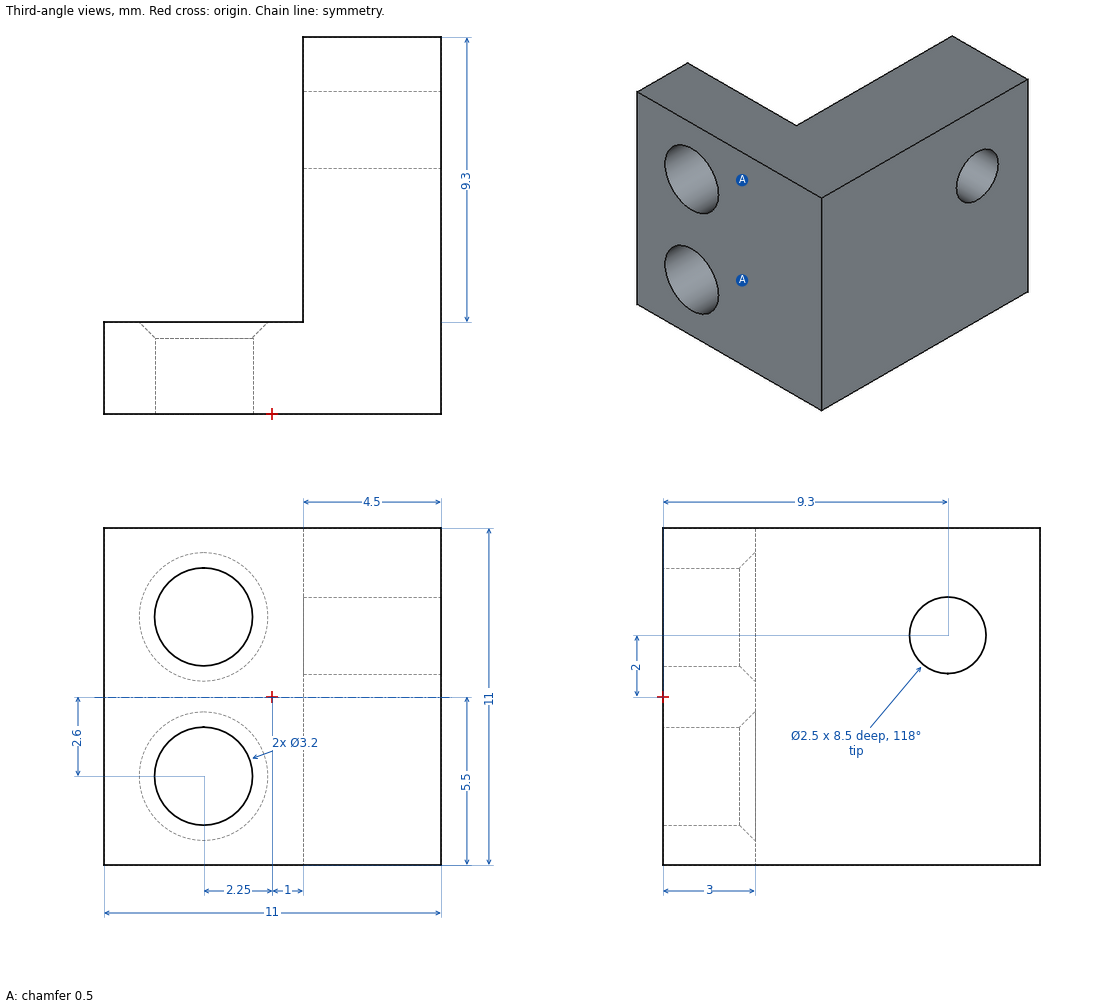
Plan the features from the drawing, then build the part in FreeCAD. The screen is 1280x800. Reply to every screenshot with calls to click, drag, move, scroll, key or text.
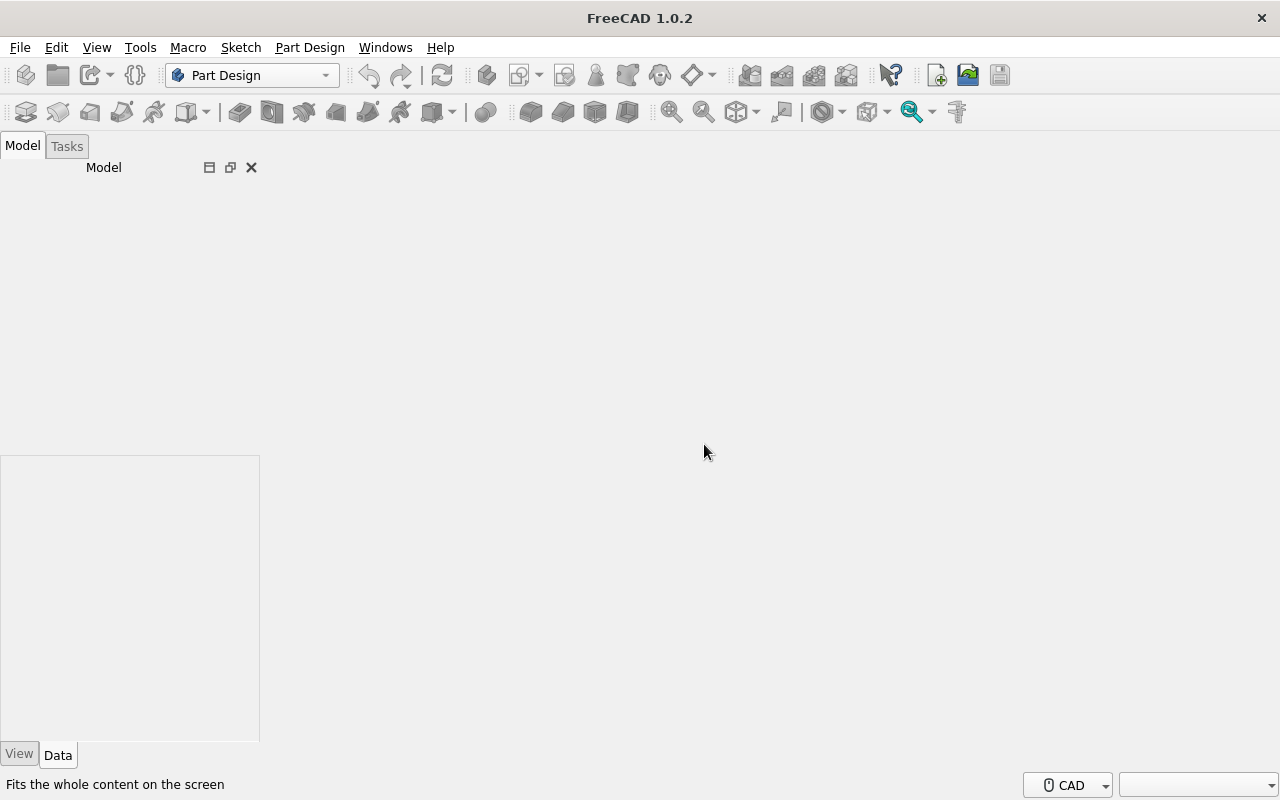
click(936, 76)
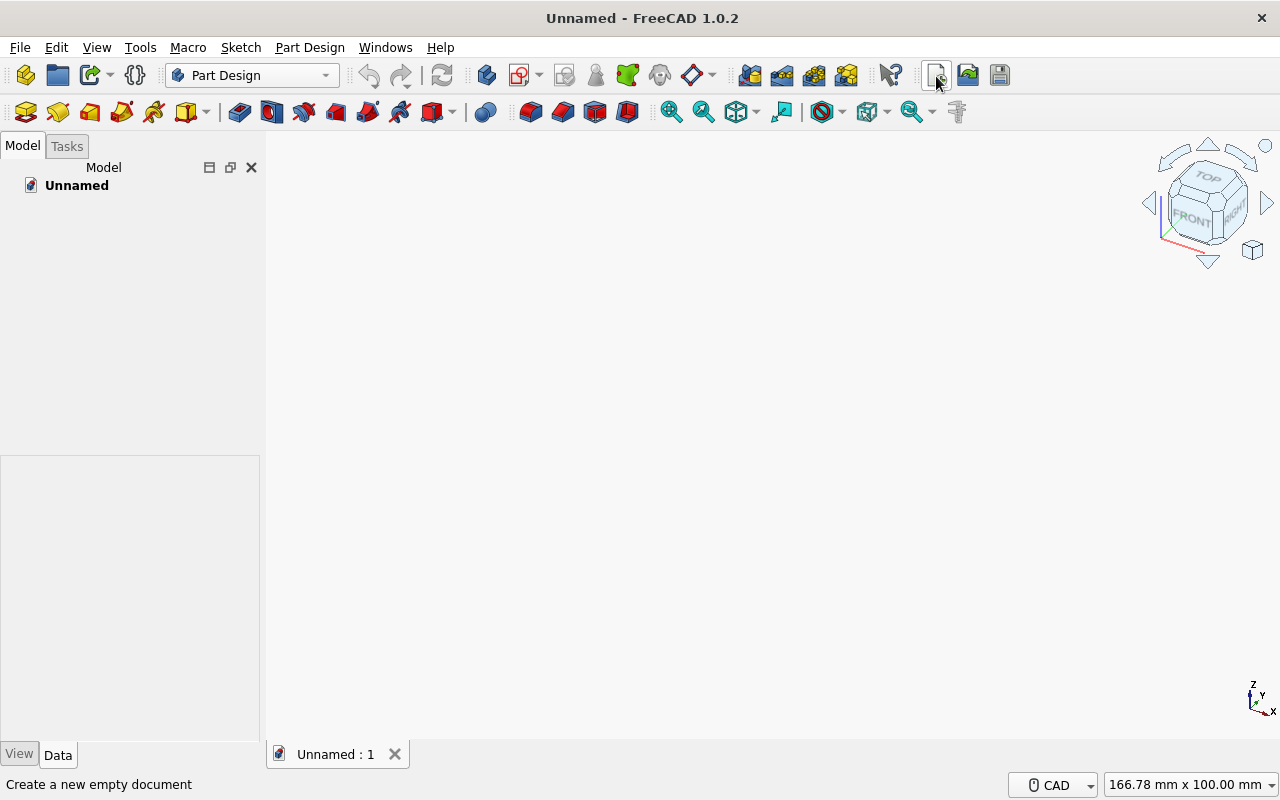
click(520, 76)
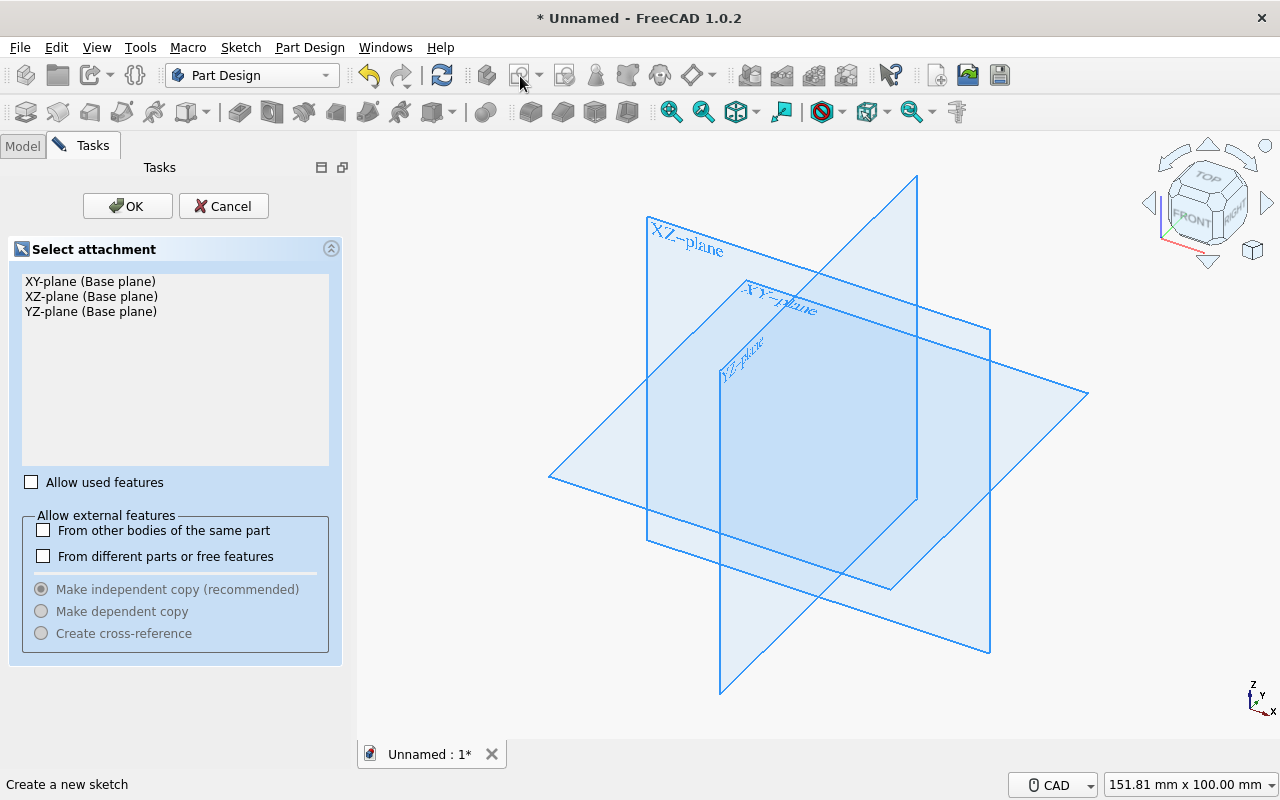
click(82, 296)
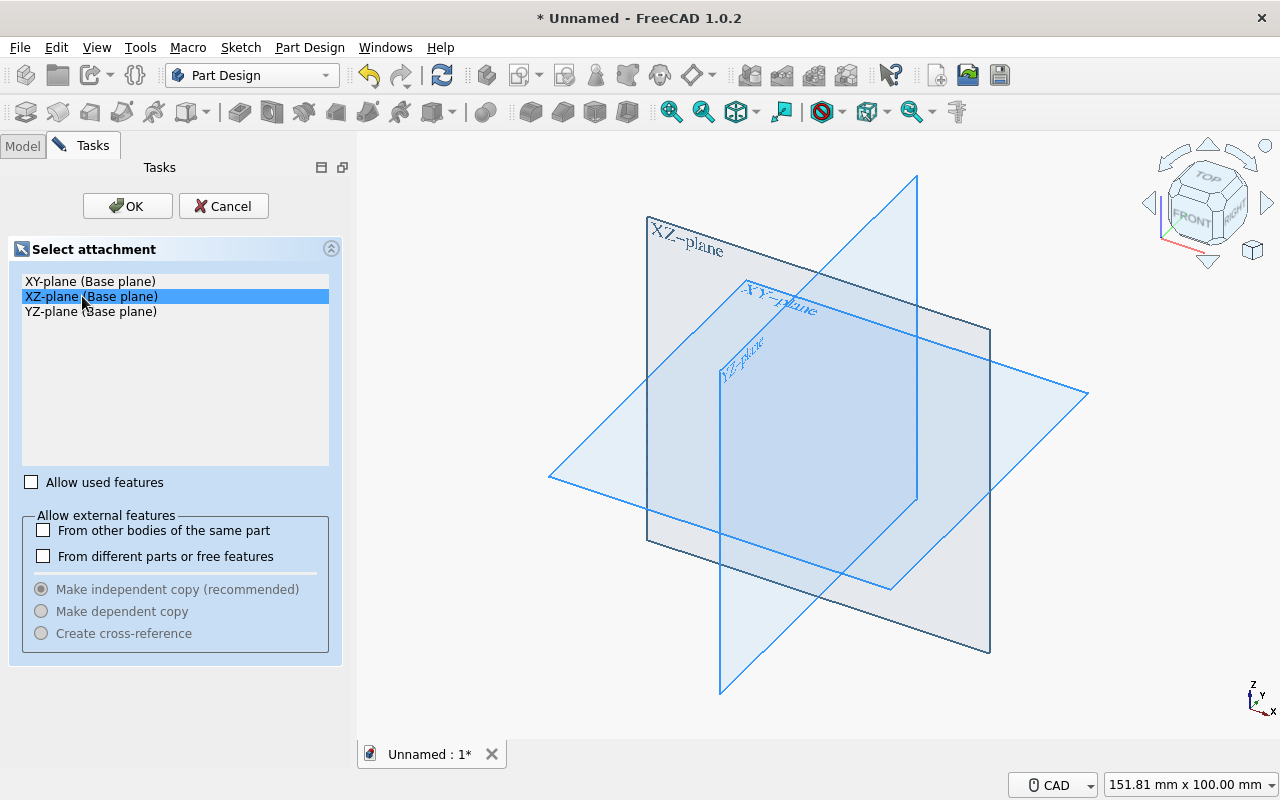
click(128, 206)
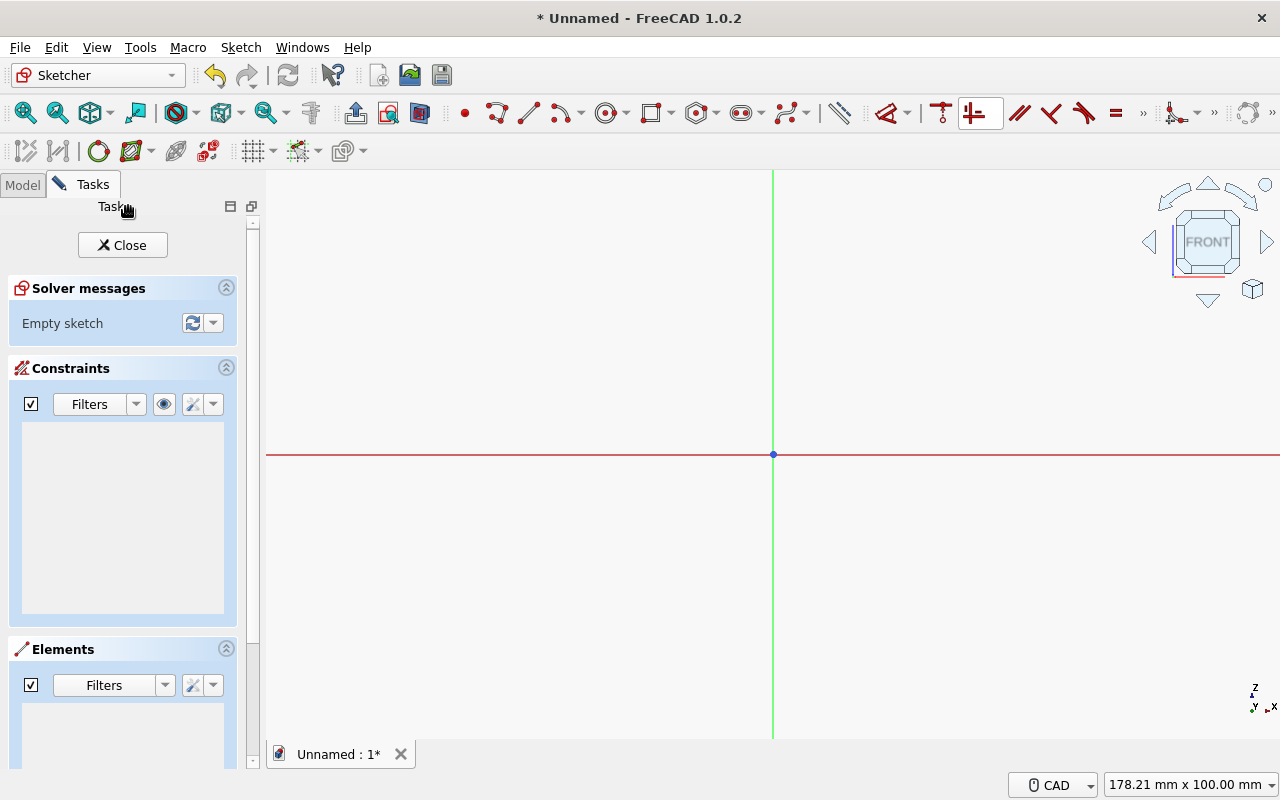
scroll(787, 455, up, 9)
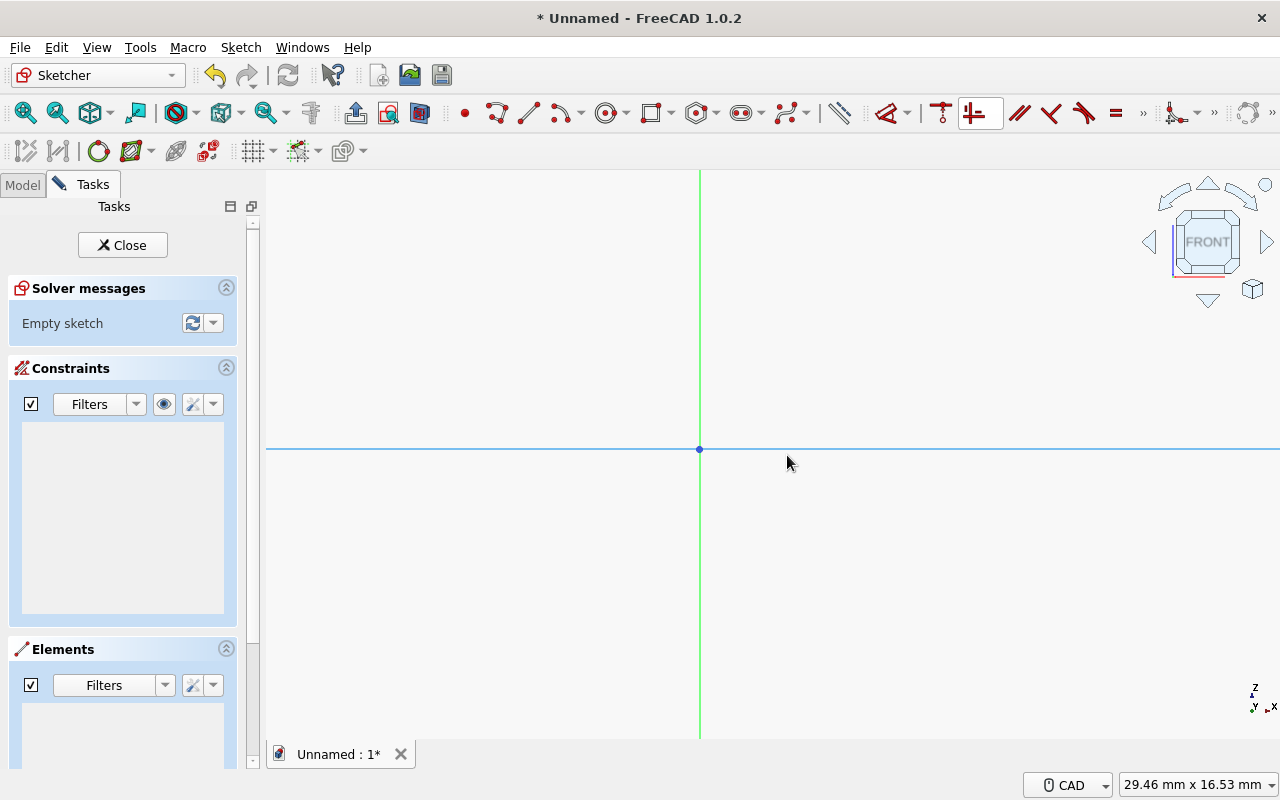
click(674, 114)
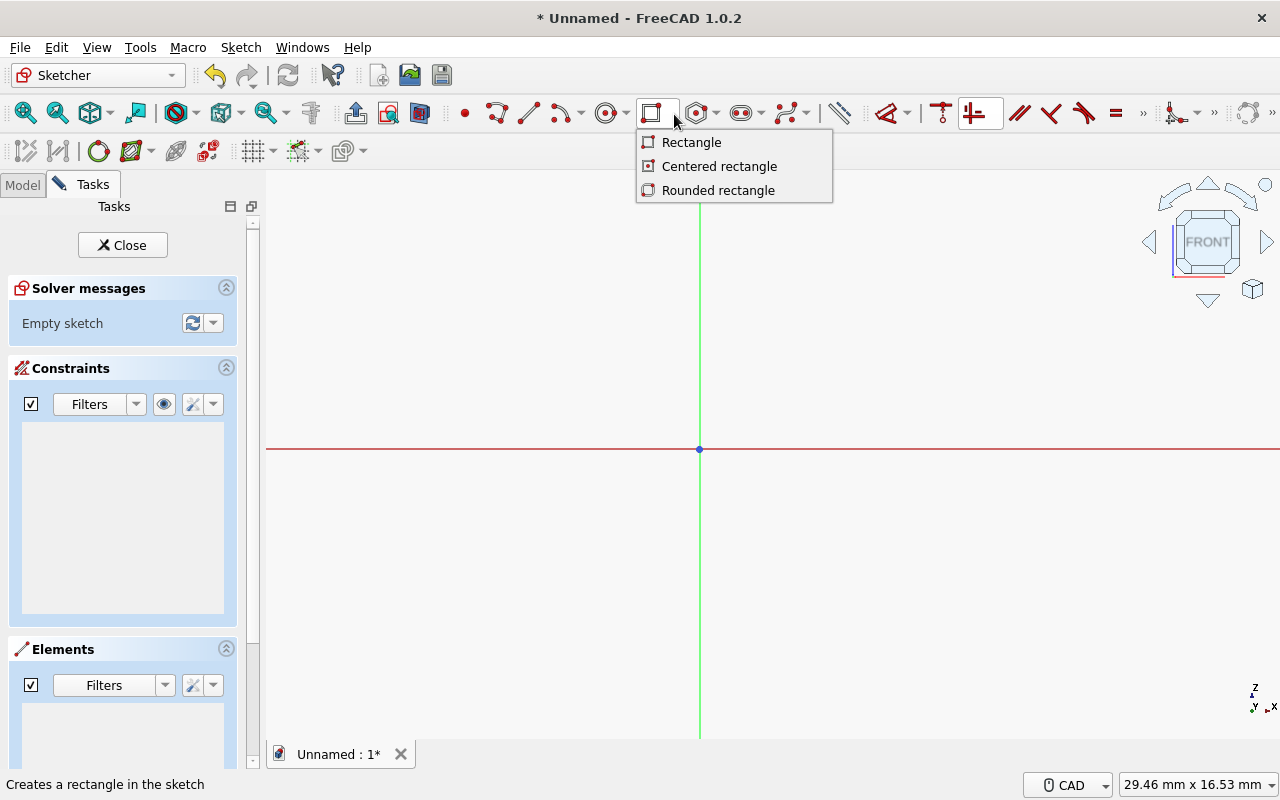
click(734, 166)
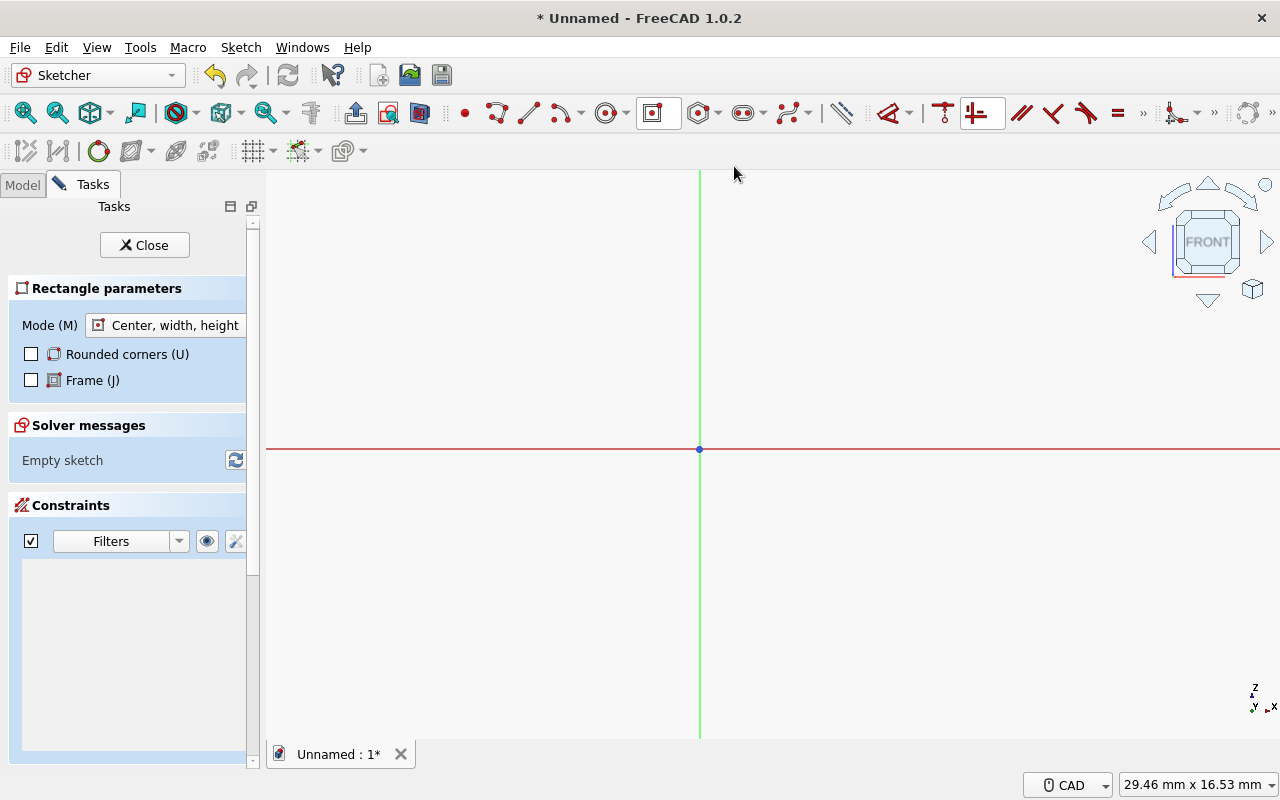
click(700, 449)
click(889, 260)
key(Escape)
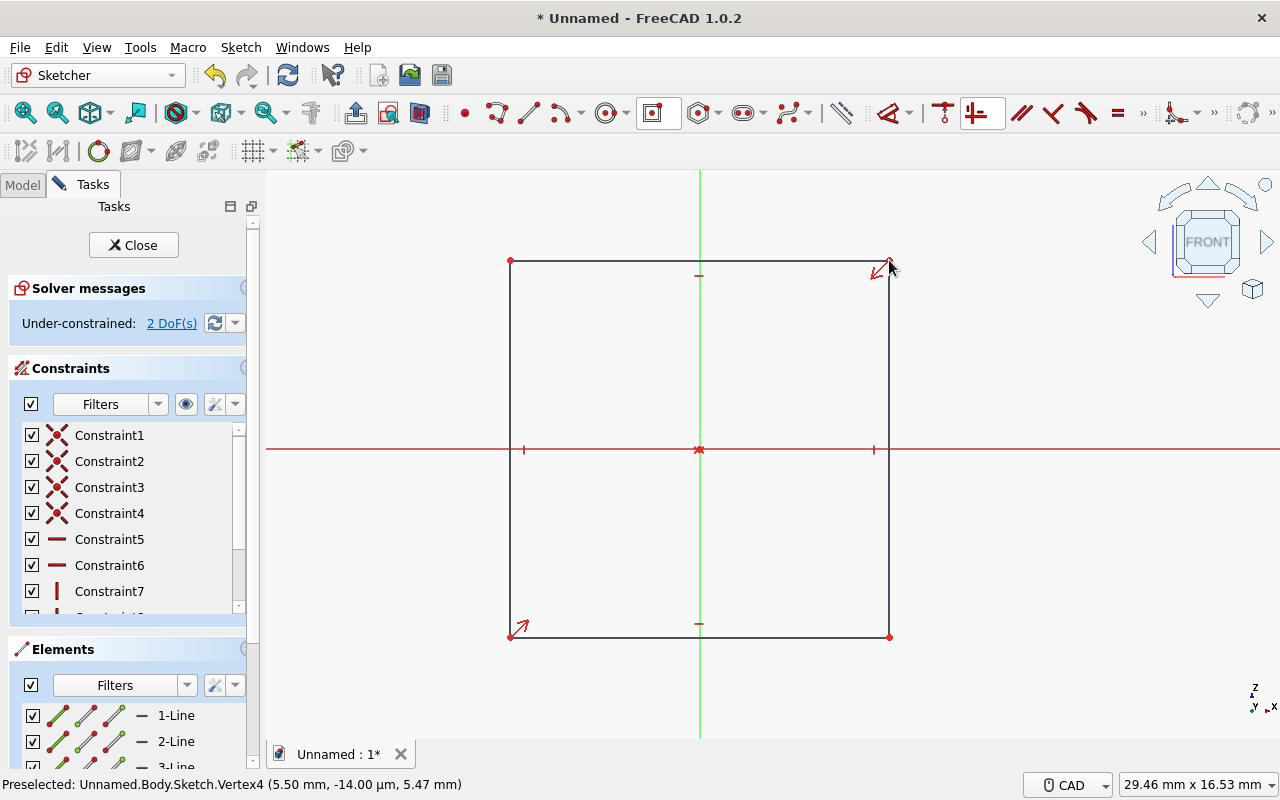
click(888, 114)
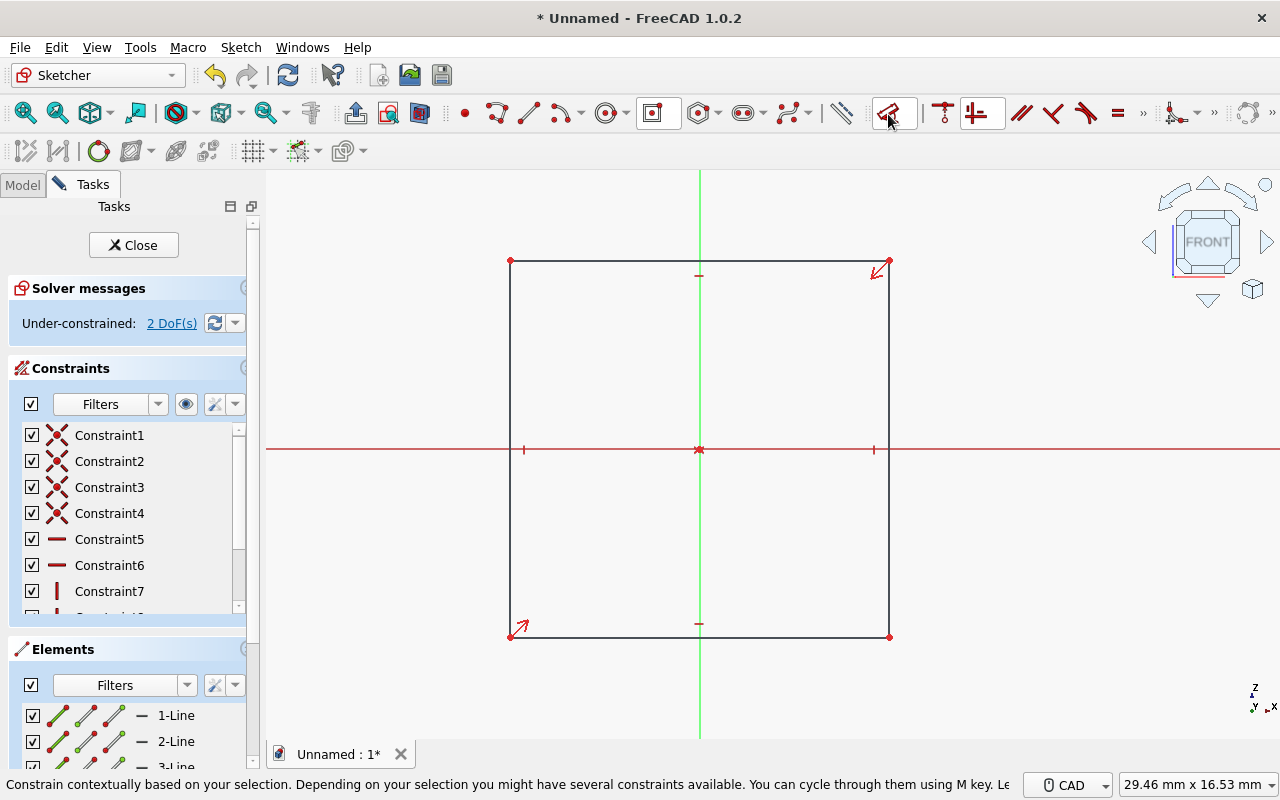
click(624, 638)
click(613, 672)